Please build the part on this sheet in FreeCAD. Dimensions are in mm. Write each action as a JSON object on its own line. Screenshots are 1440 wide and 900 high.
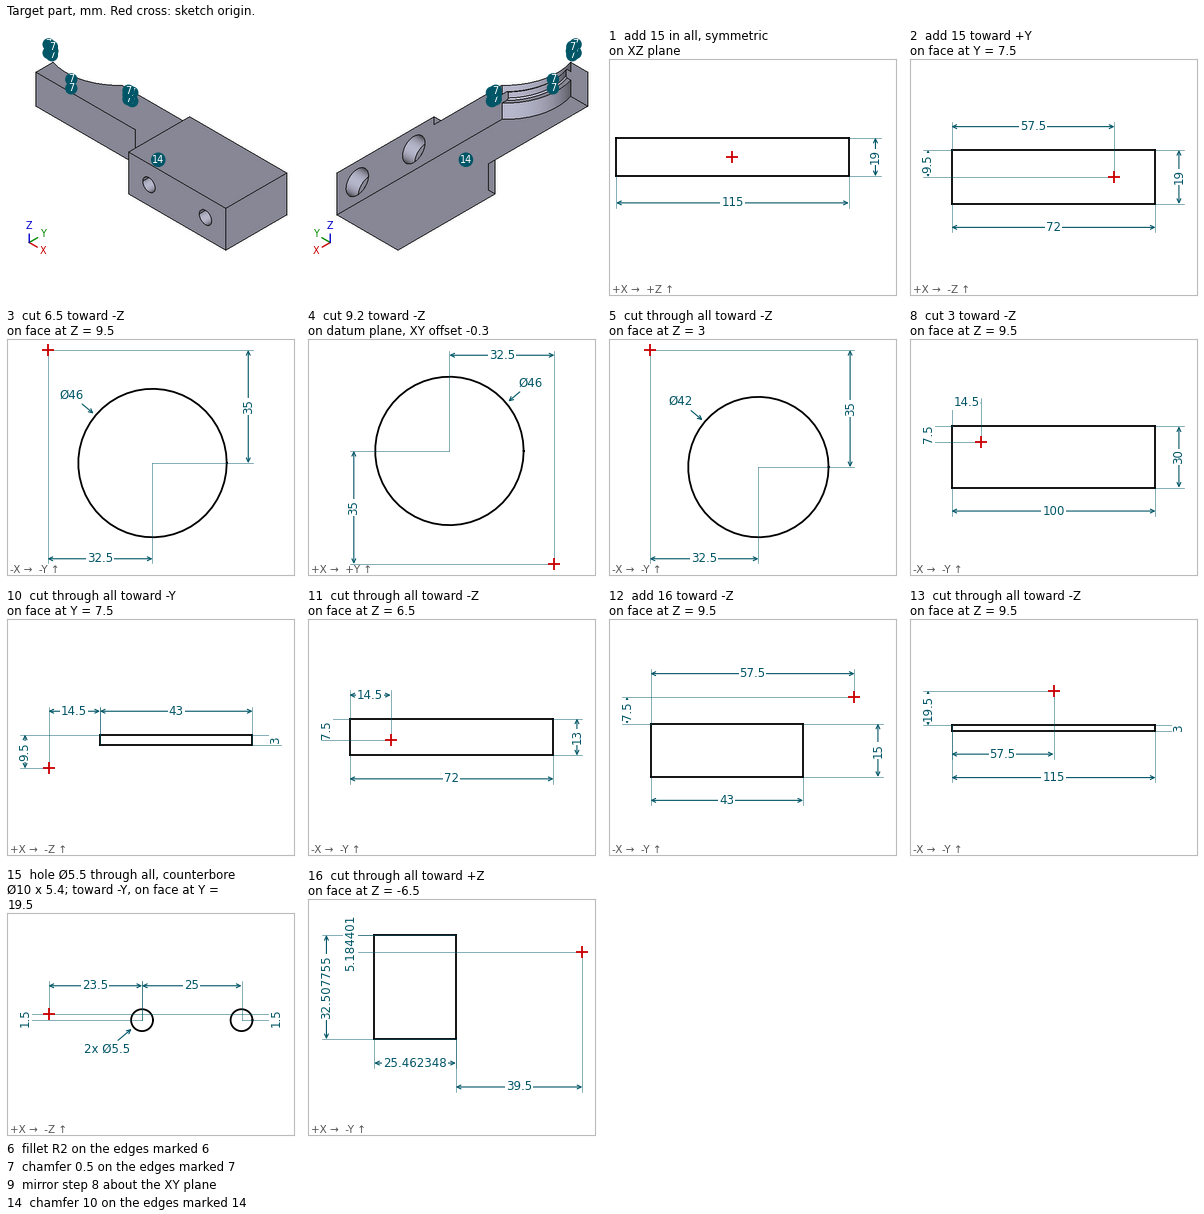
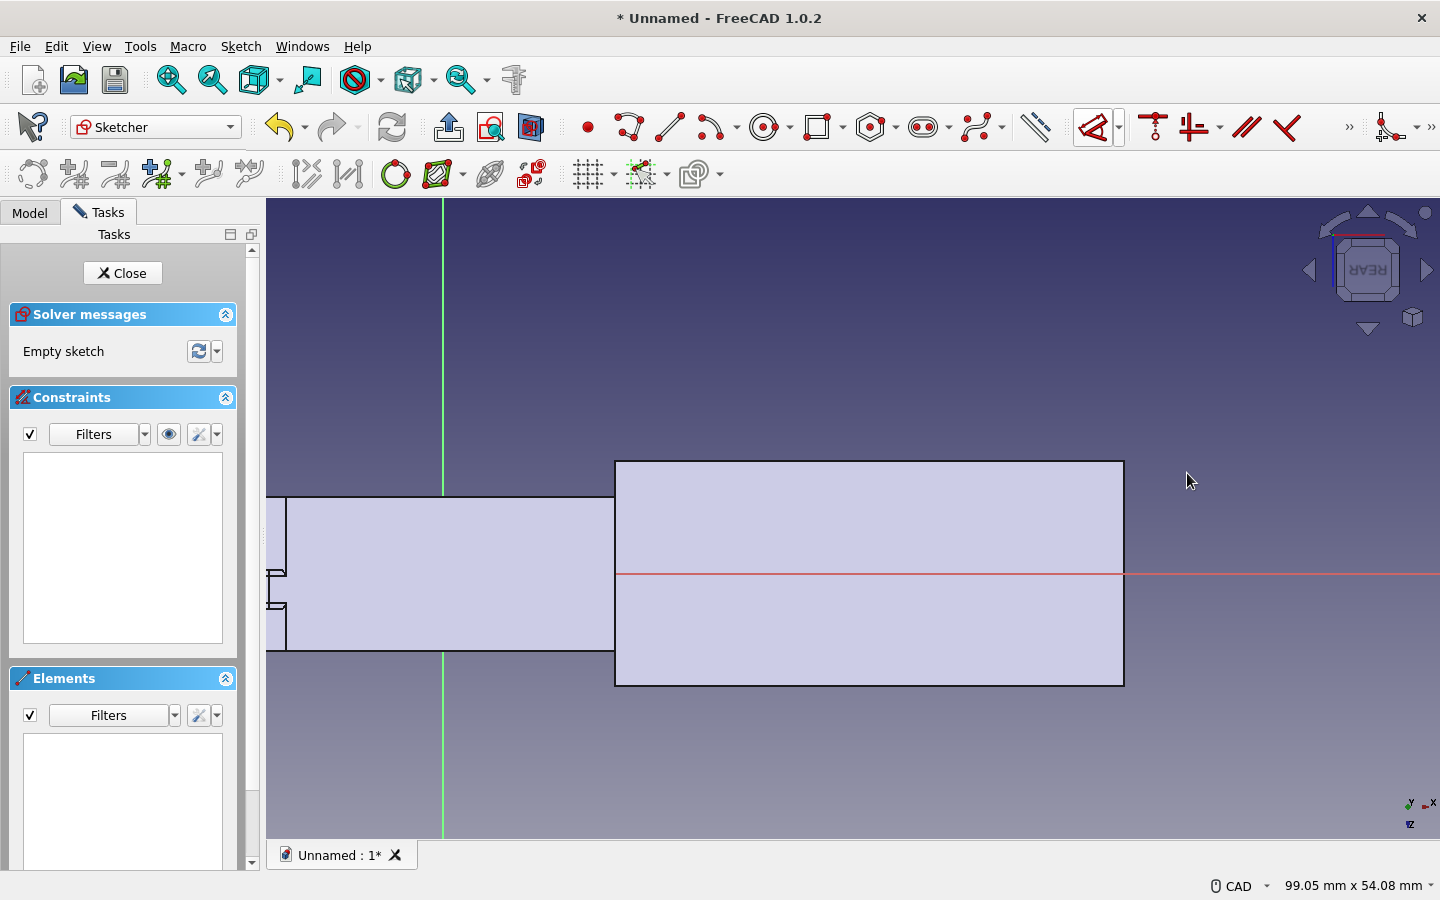
{"action": "left_click", "coordinate": [816, 128]}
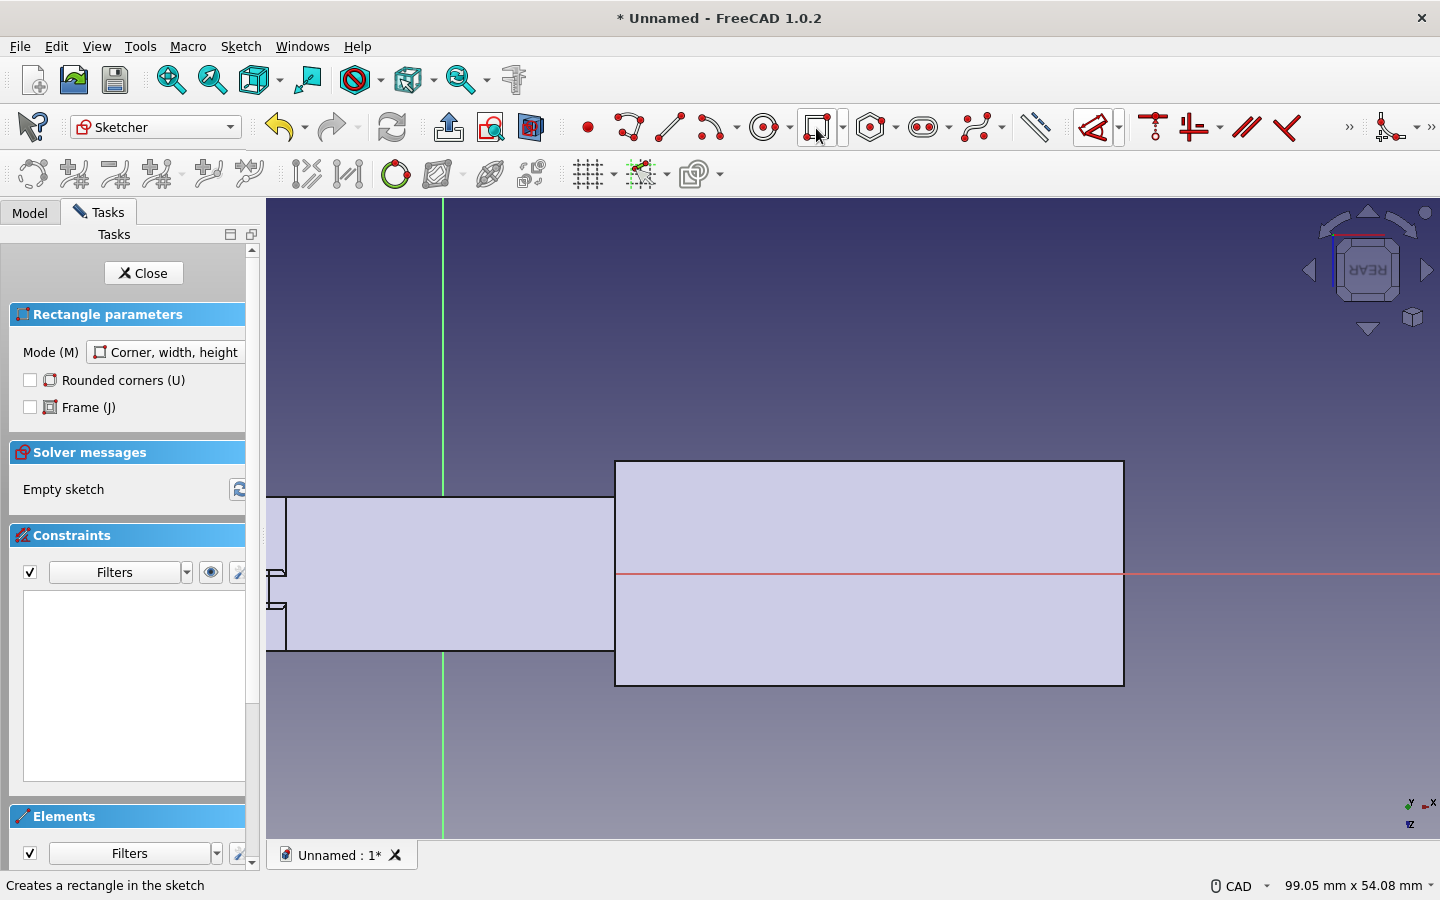
{"action": "left_click", "coordinate": [615, 461]}
{"action": "mouse_move", "coordinate": [1124, 497]}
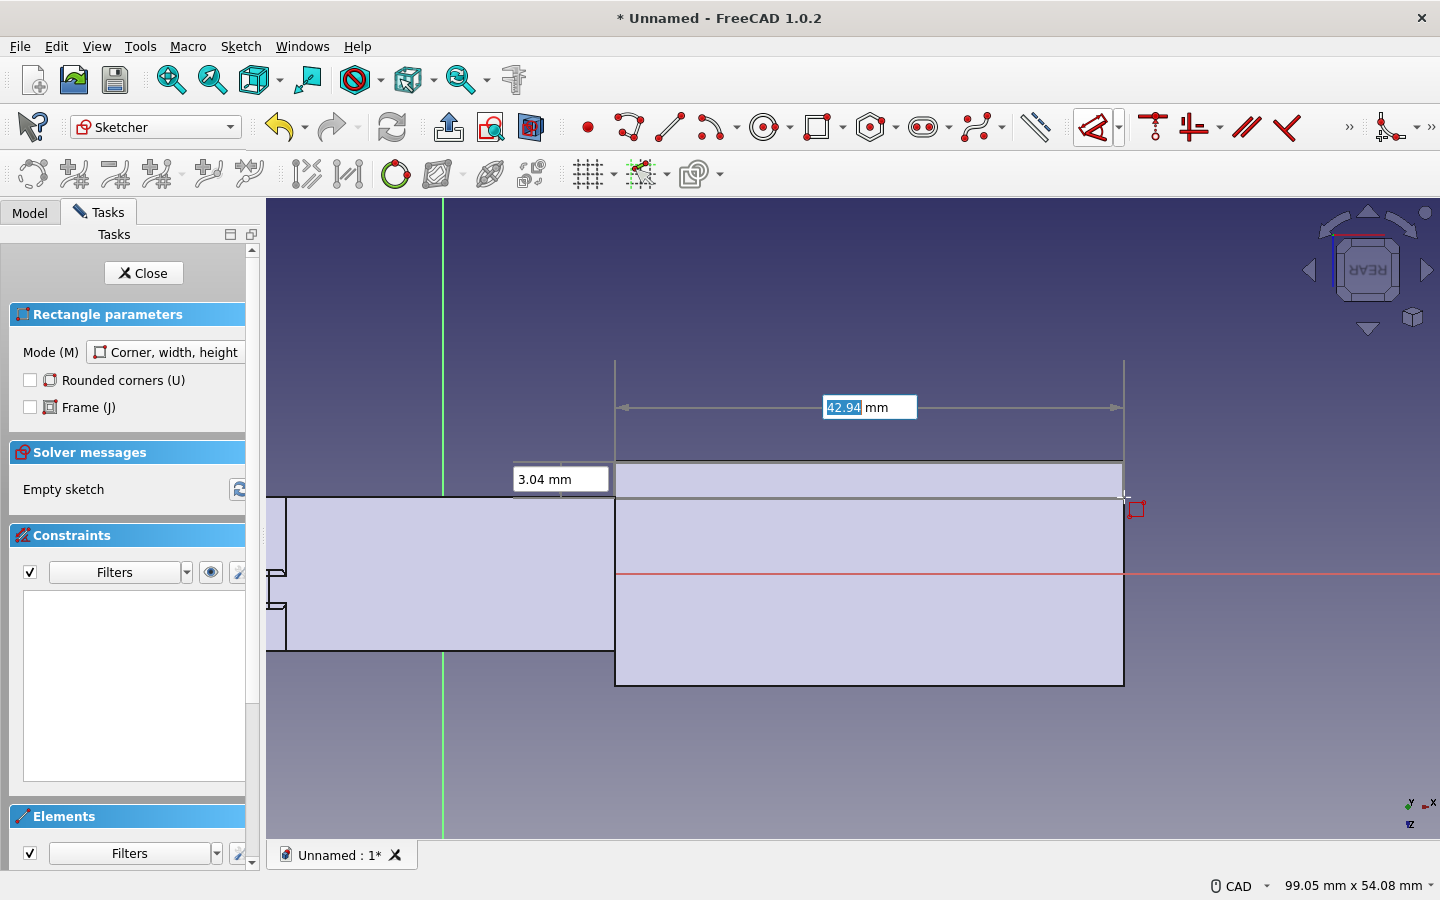
{"action": "type", "text": "43"}
{"action": "key", "text": "Tab"}
{"action": "type", "text": "3"}
{"action": "key", "text": "Return"}
{"action": "key", "text": "Escape"}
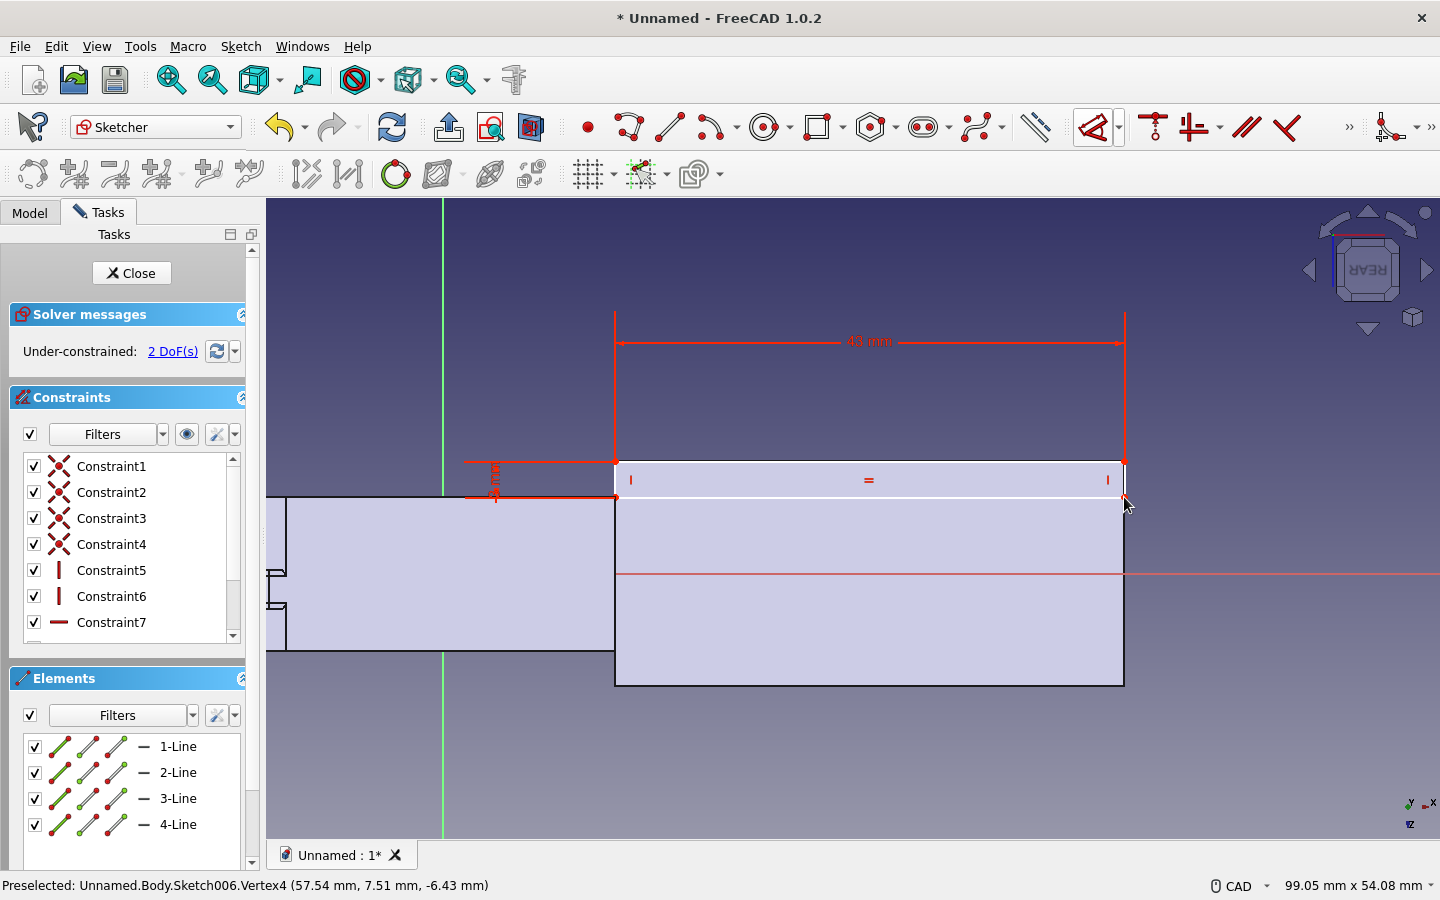
{"action": "left_click", "coordinate": [615, 462]}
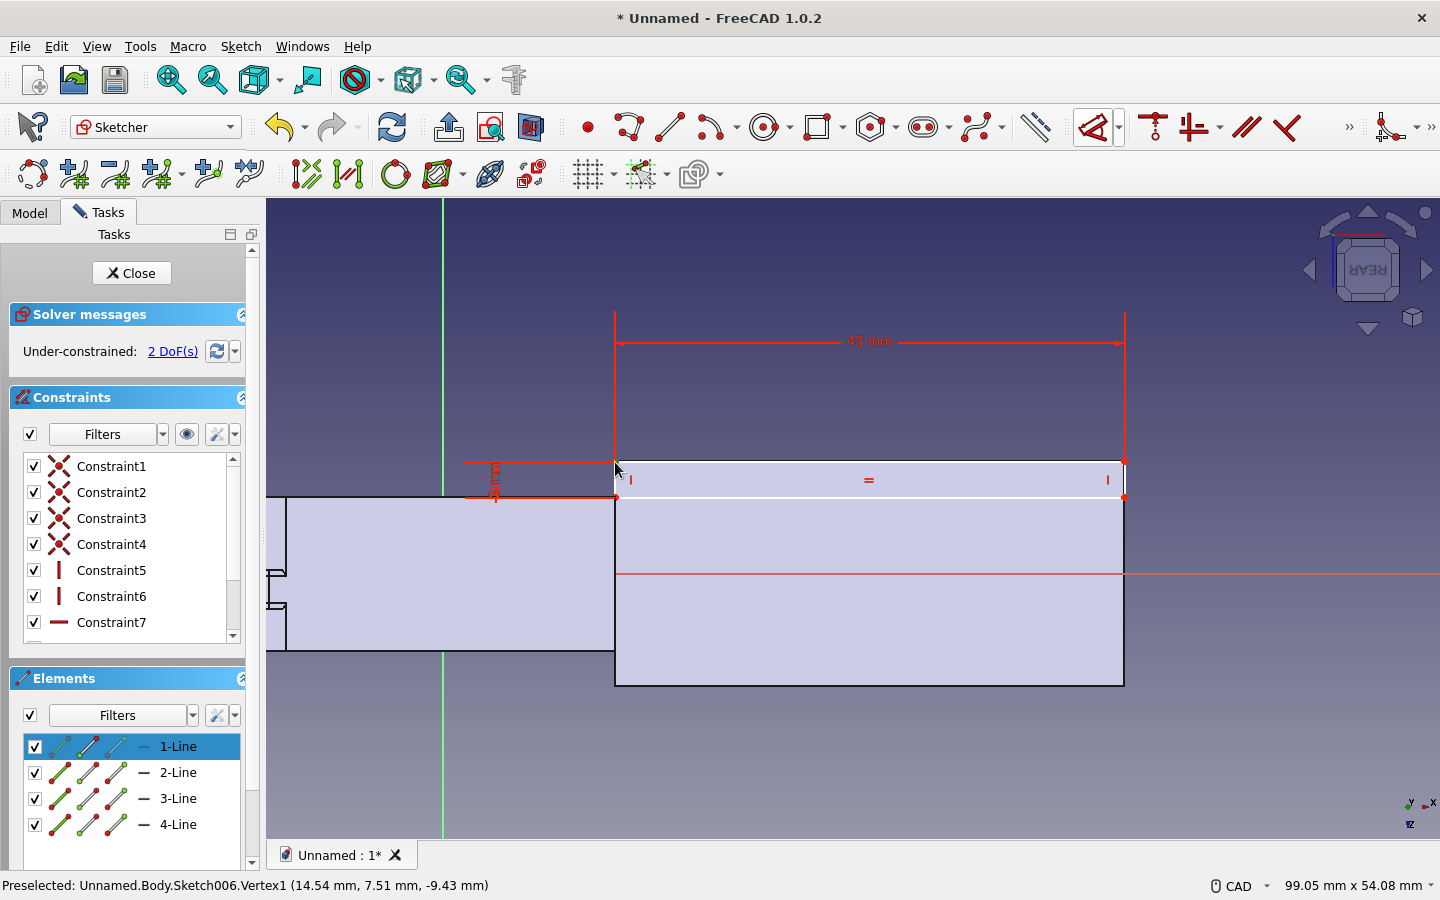
{"action": "left_click", "coordinate": [1118, 128]}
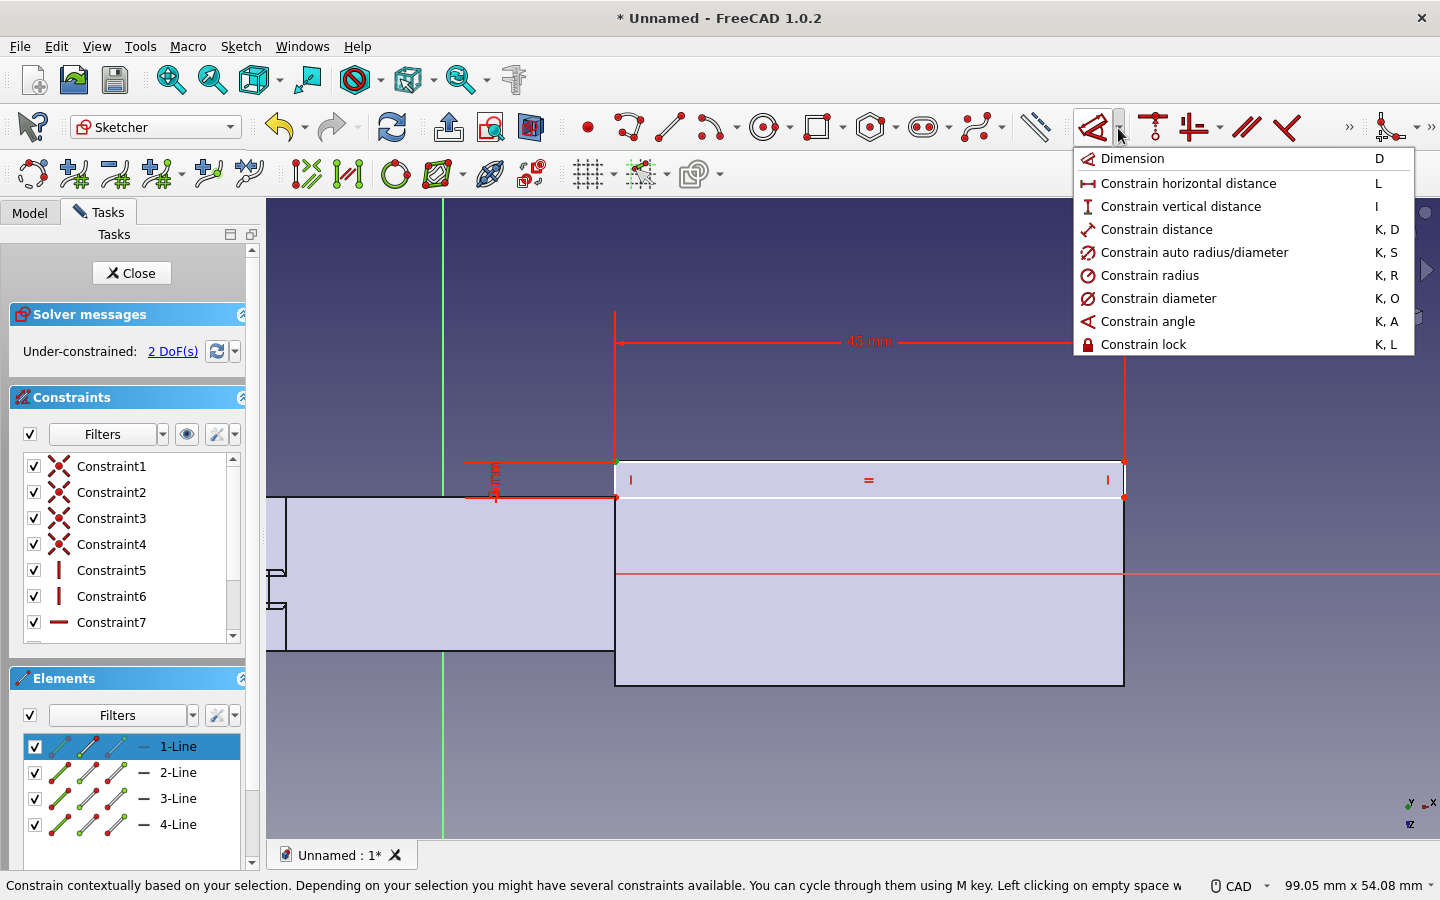
{"action": "left_click", "coordinate": [1244, 206]}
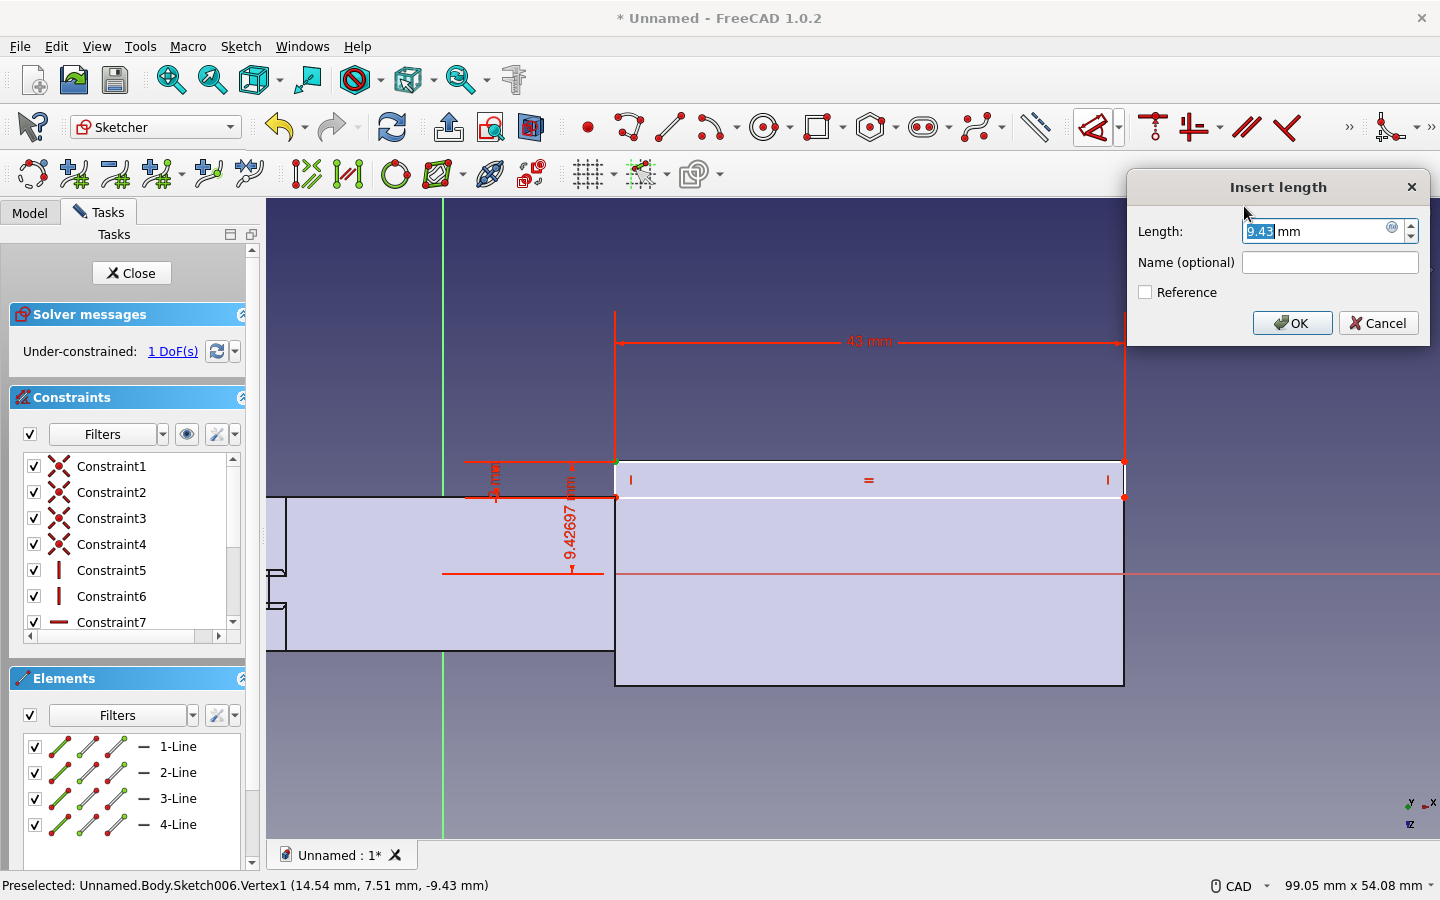
{"action": "type", "text": "9.5"}
{"action": "key", "text": "Return"}